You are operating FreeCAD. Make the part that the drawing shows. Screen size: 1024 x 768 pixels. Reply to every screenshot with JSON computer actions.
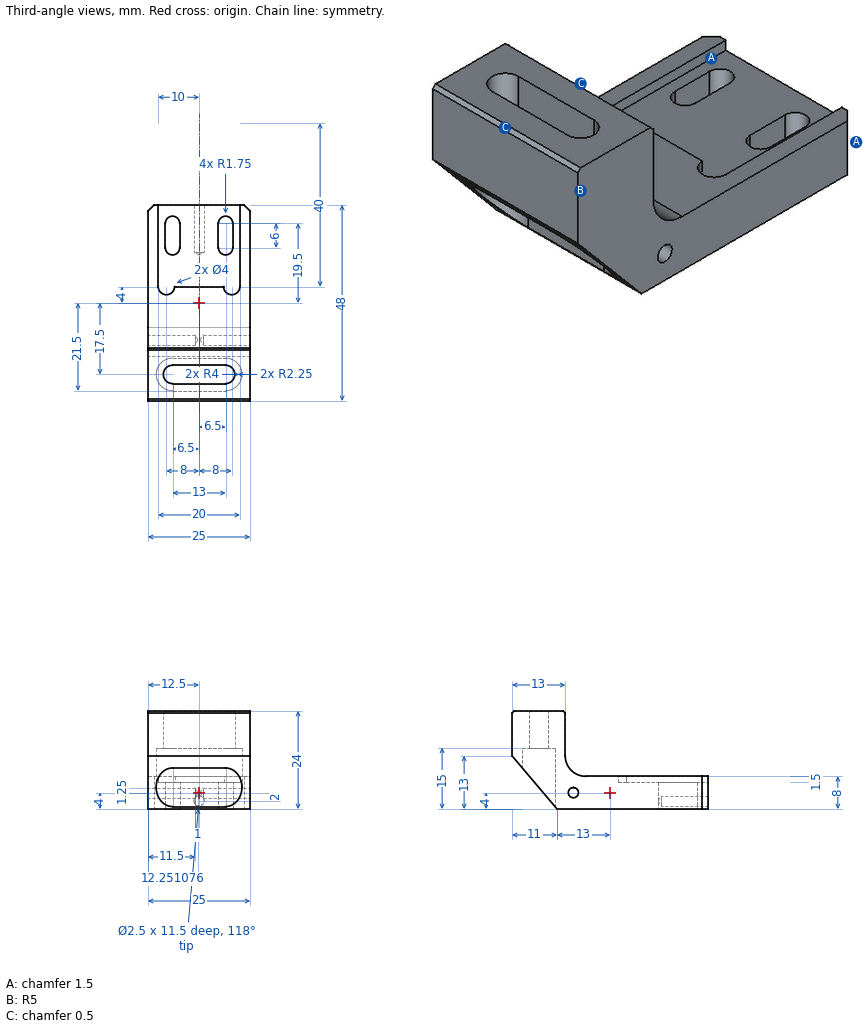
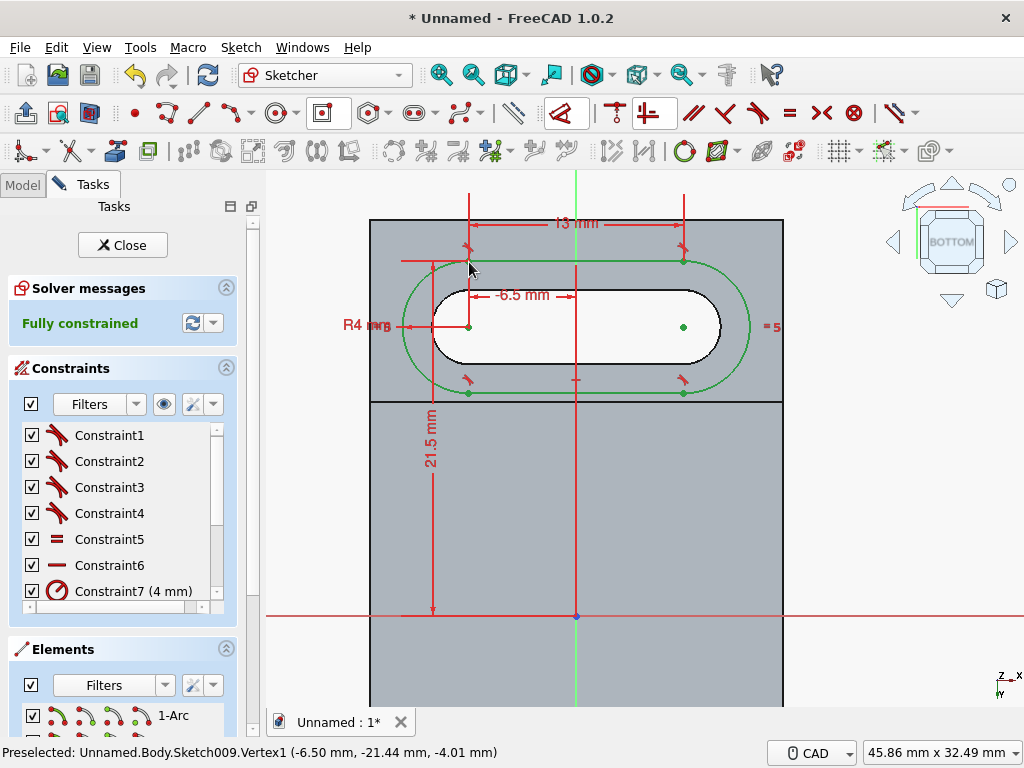
{"action": "left_click", "coordinate": [123, 245]}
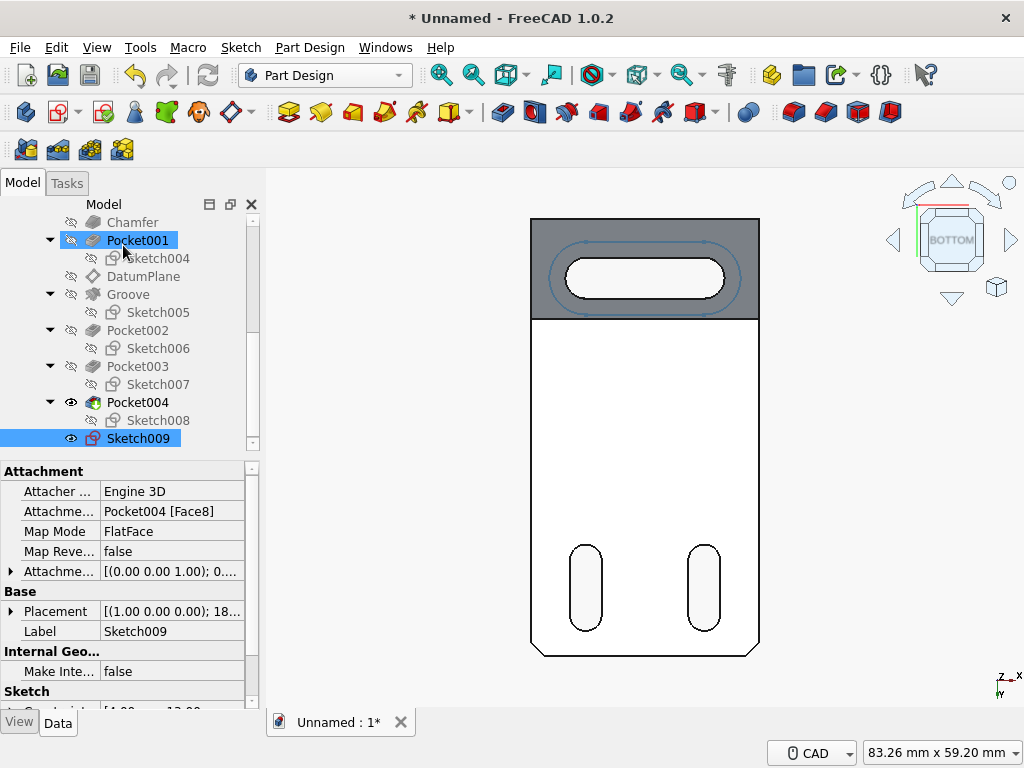
{"action": "left_click", "coordinate": [504, 112]}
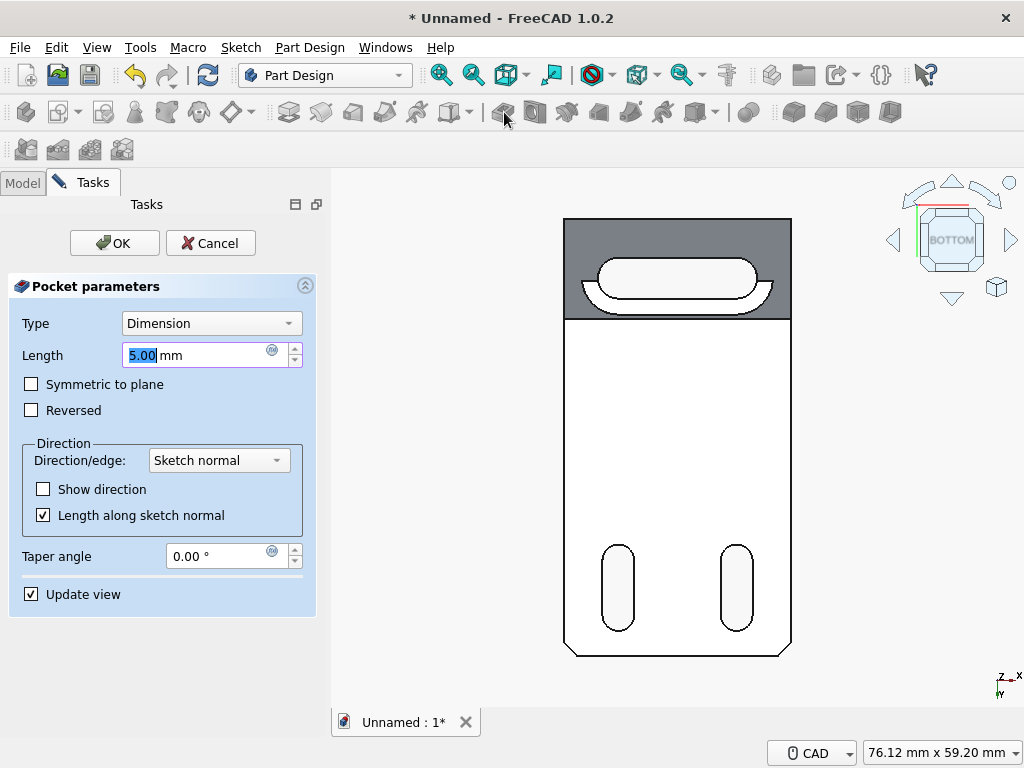
{"action": "type", "text": "15"}
{"action": "key", "text": "Tab"}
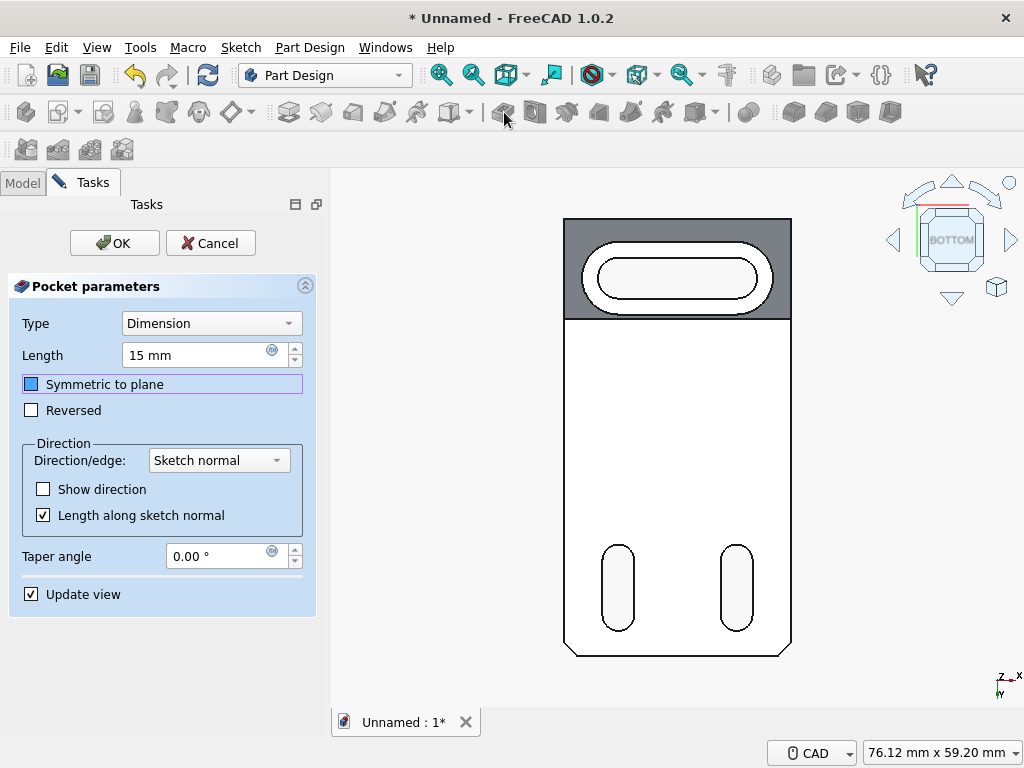
{"action": "left_click", "coordinate": [115, 243]}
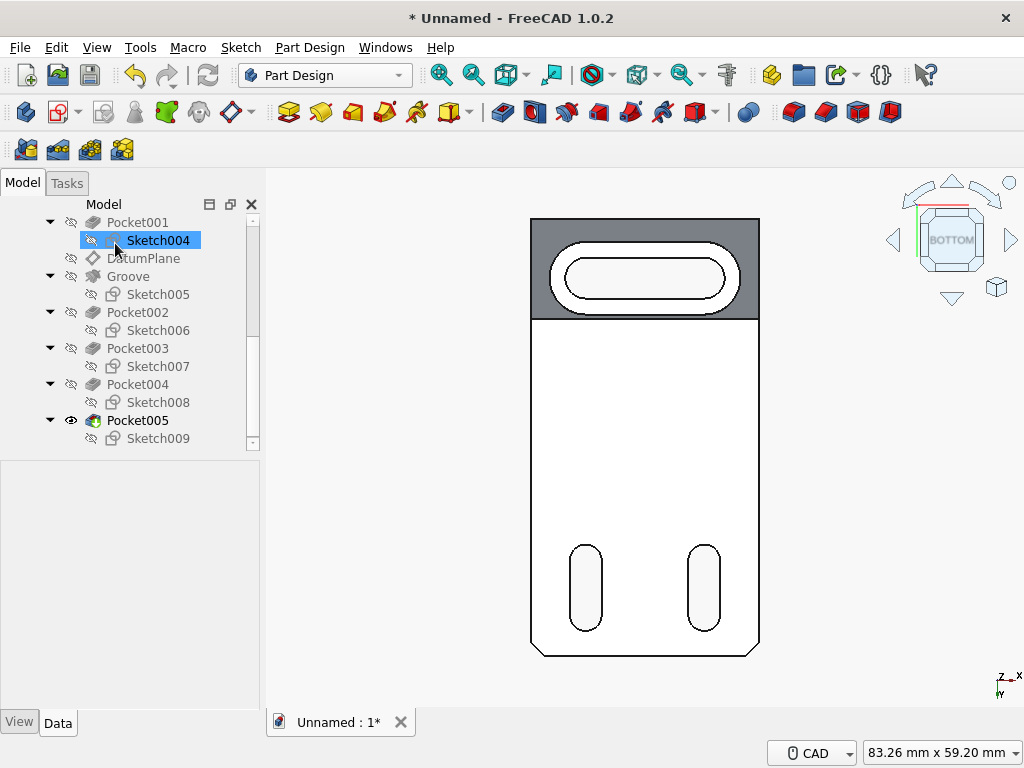
{"action": "key", "text": "0"}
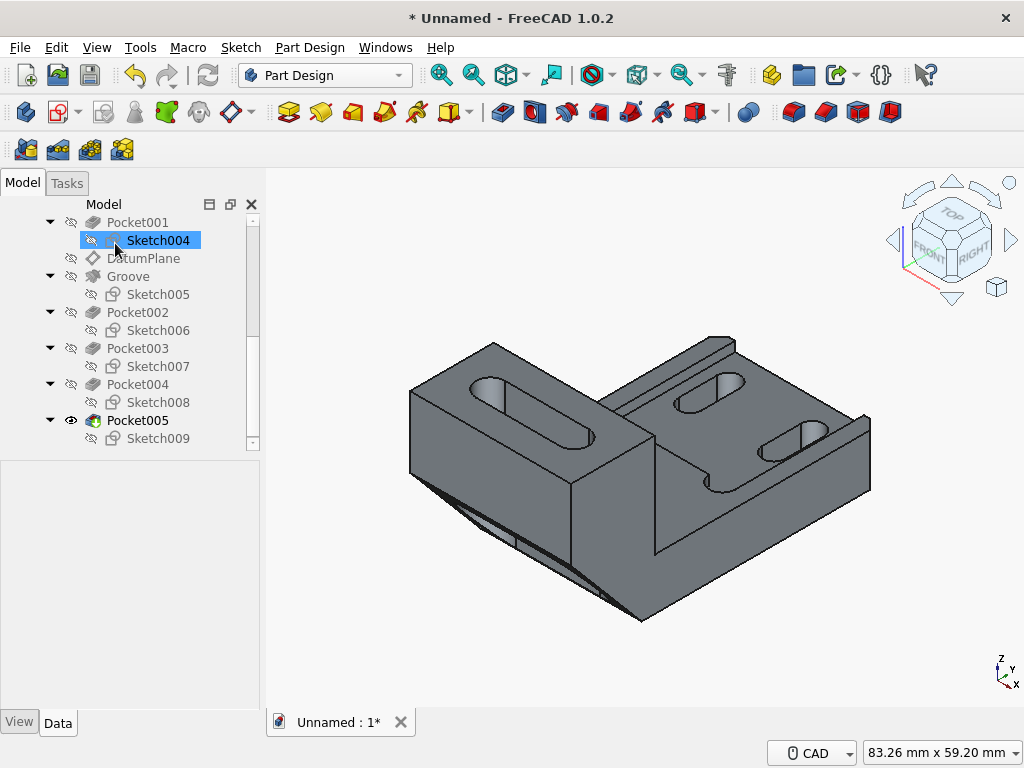
{"action": "key", "text": "2"}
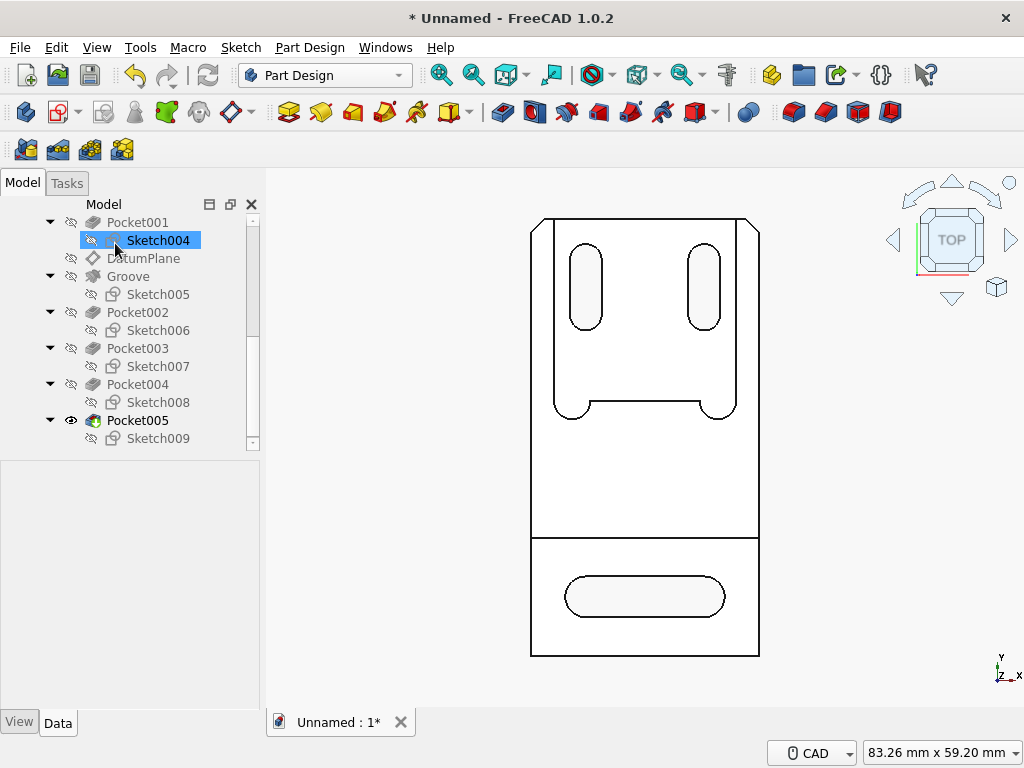
{"action": "key", "text": "1"}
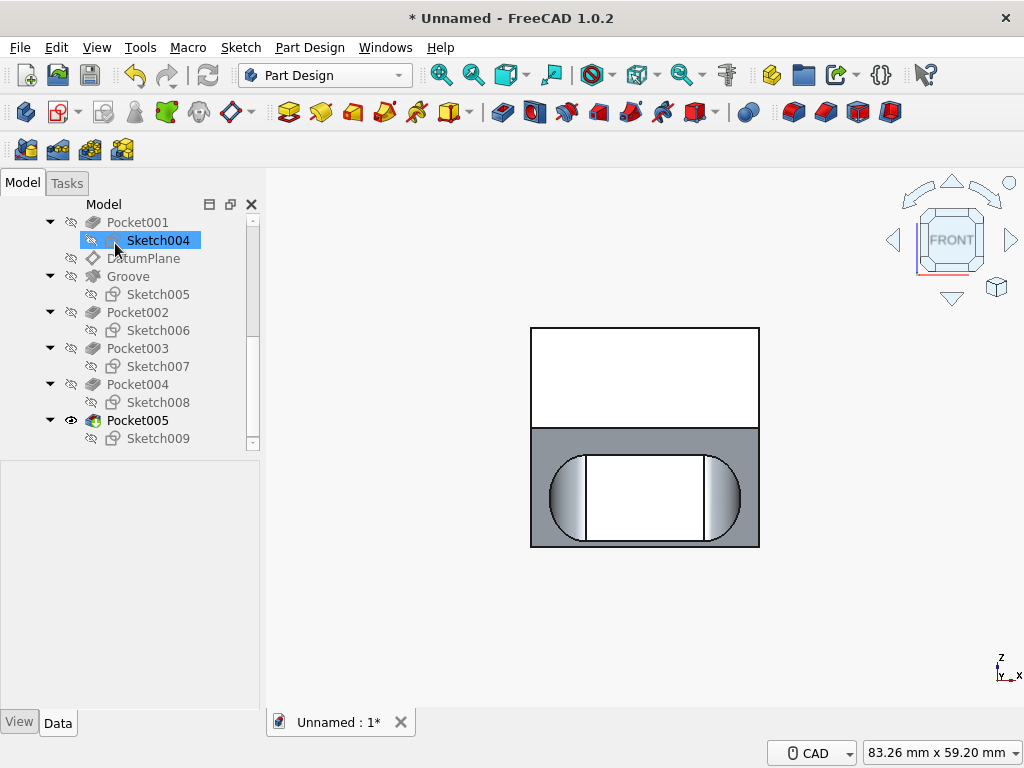
{"action": "left_click", "coordinate": [442, 76]}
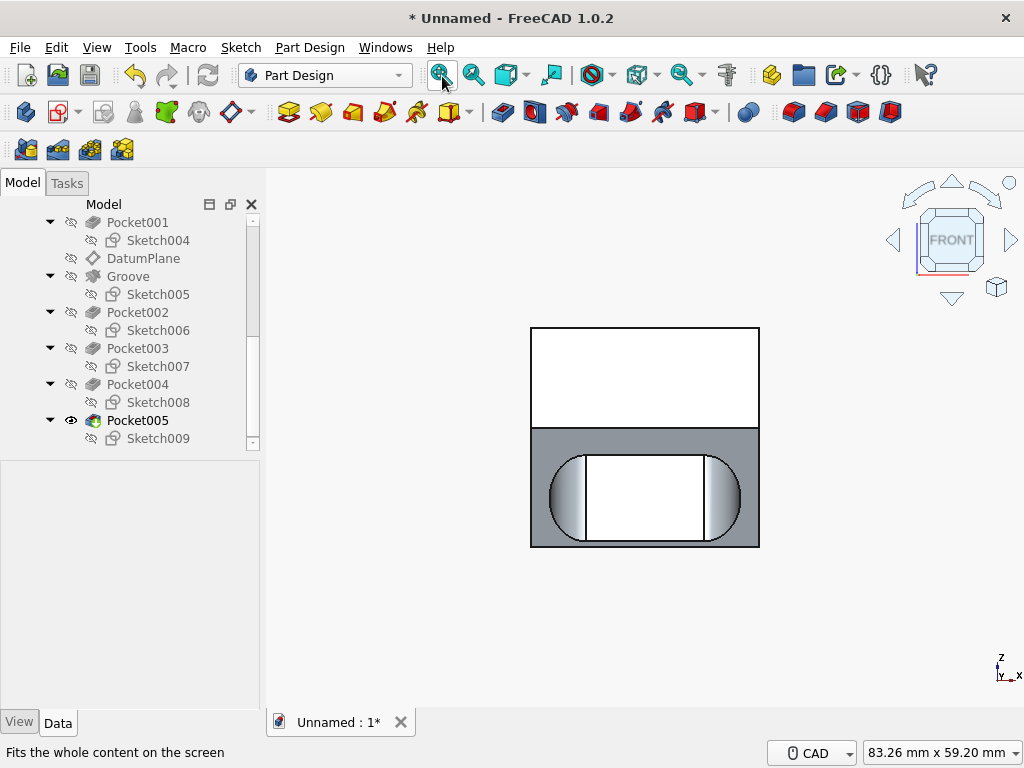
{"action": "key", "text": "3"}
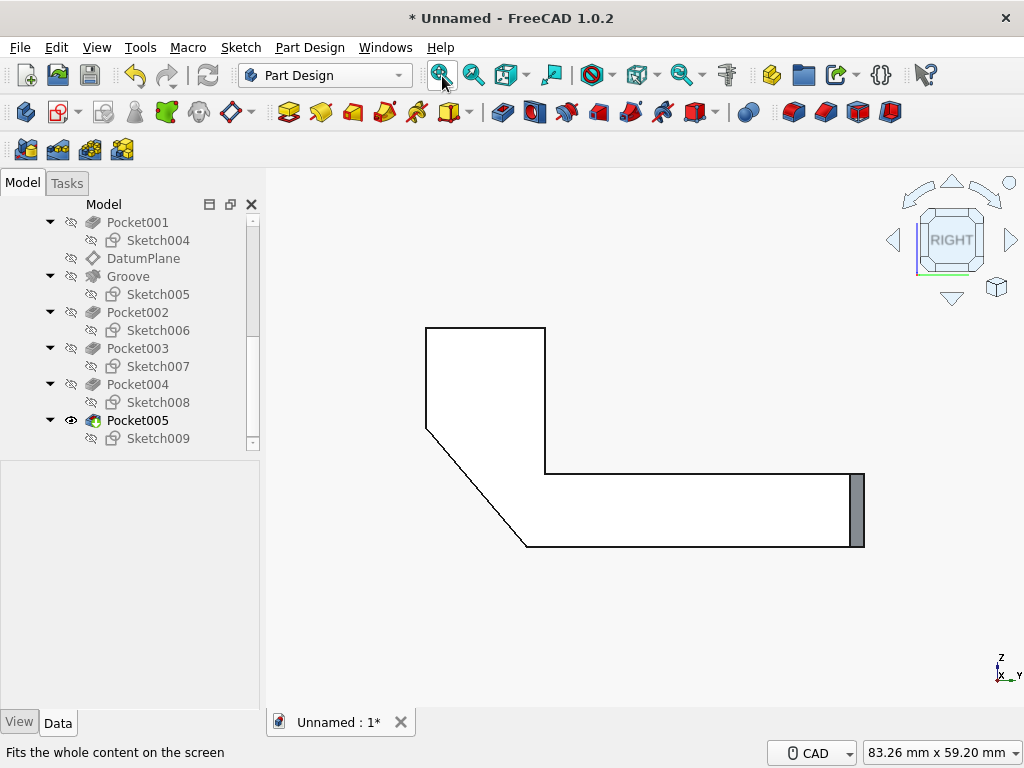
{"action": "key", "text": "5"}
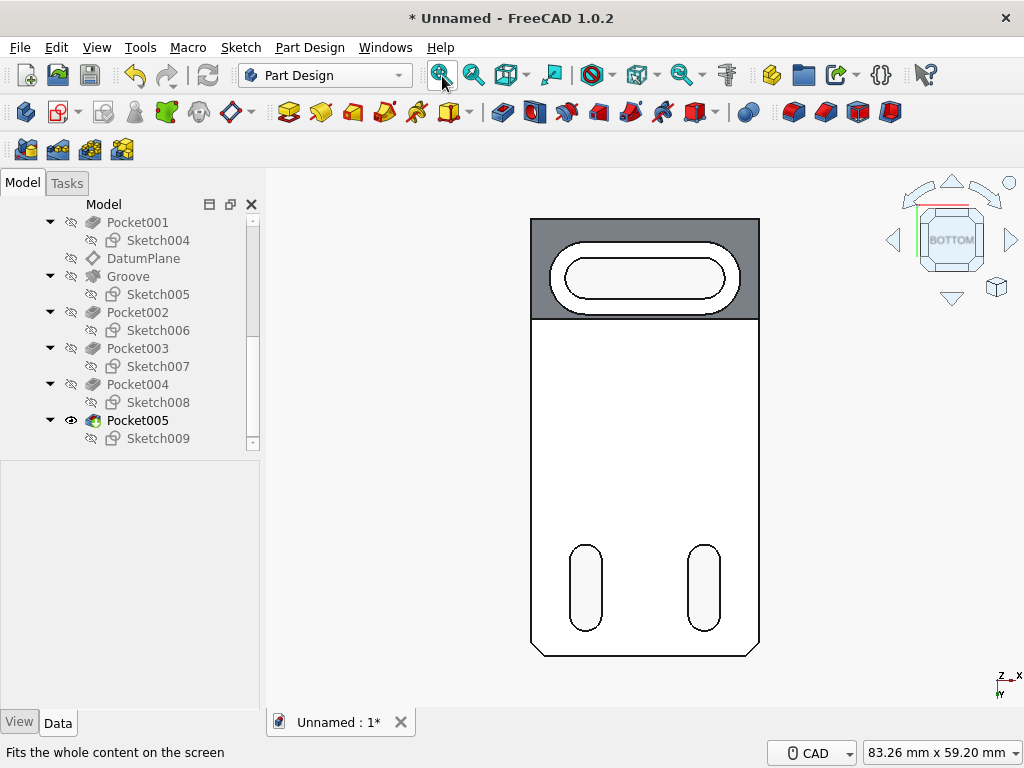
{"action": "key", "text": "4"}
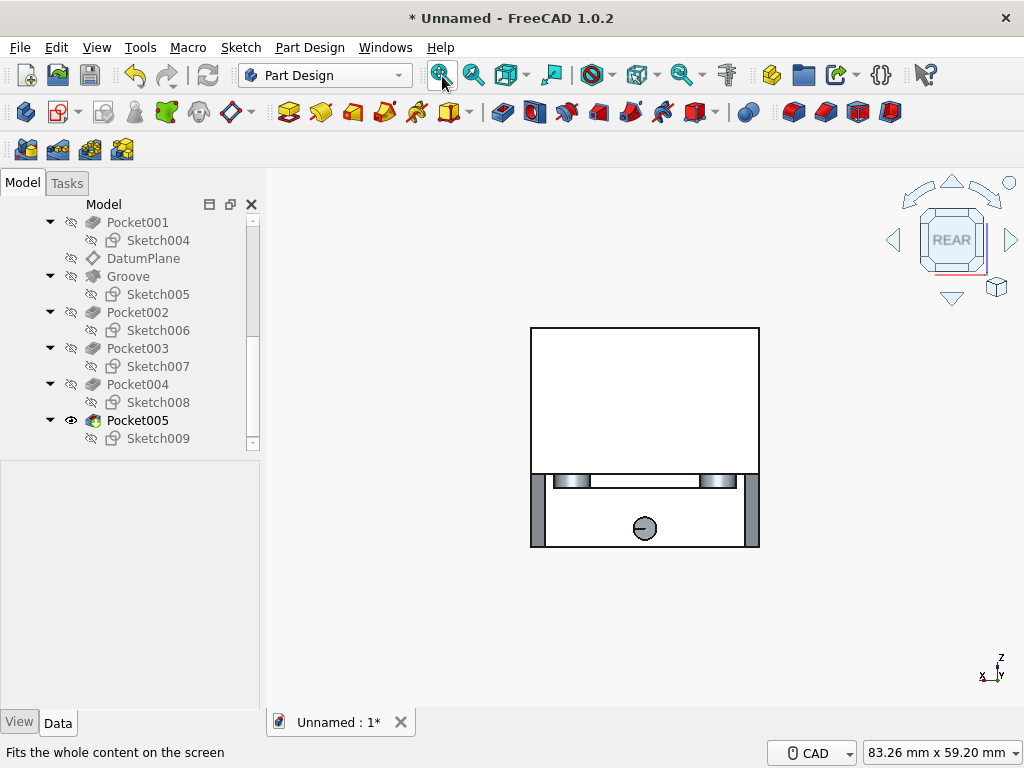
{"action": "left_click", "coordinate": [442, 76]}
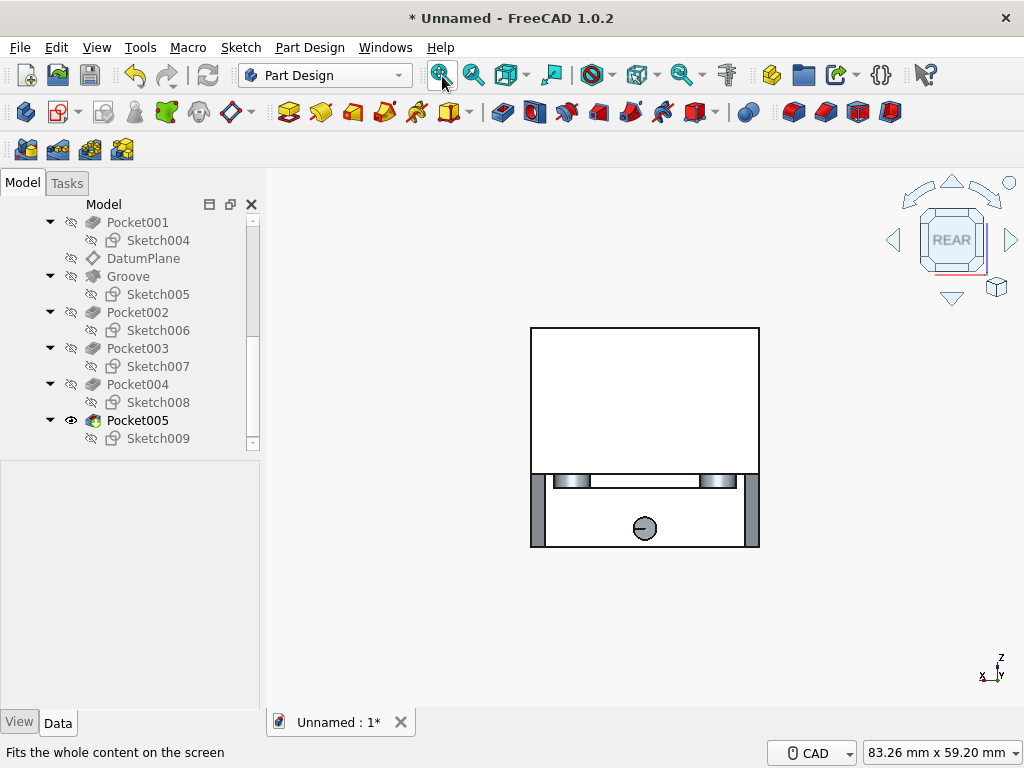
{"action": "key", "text": "6"}